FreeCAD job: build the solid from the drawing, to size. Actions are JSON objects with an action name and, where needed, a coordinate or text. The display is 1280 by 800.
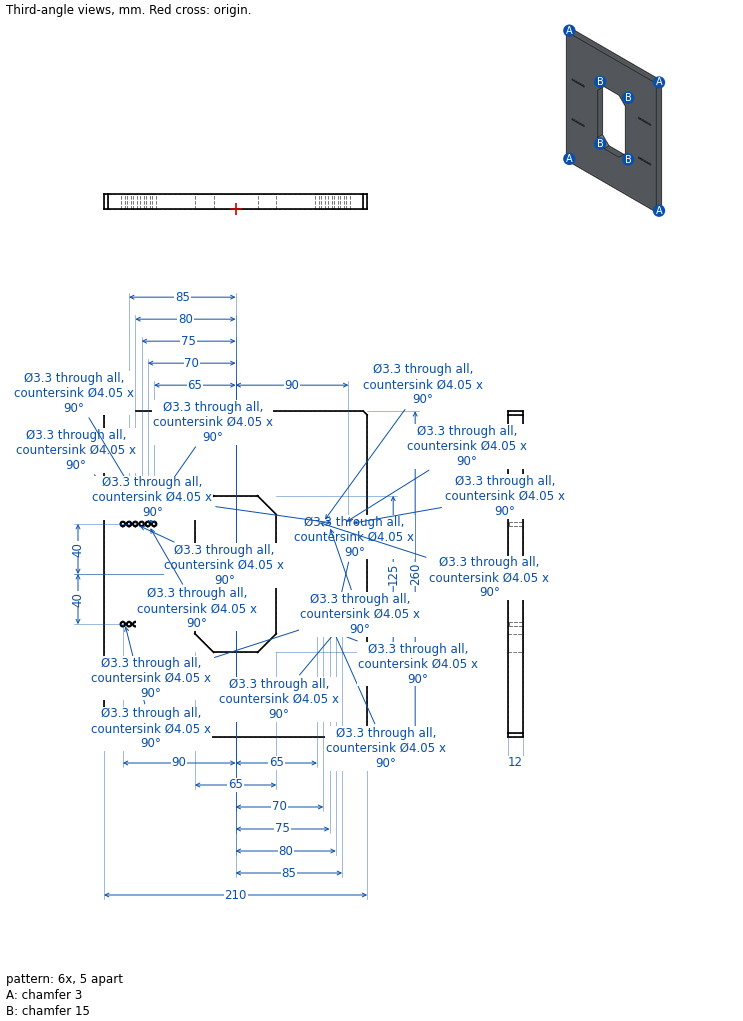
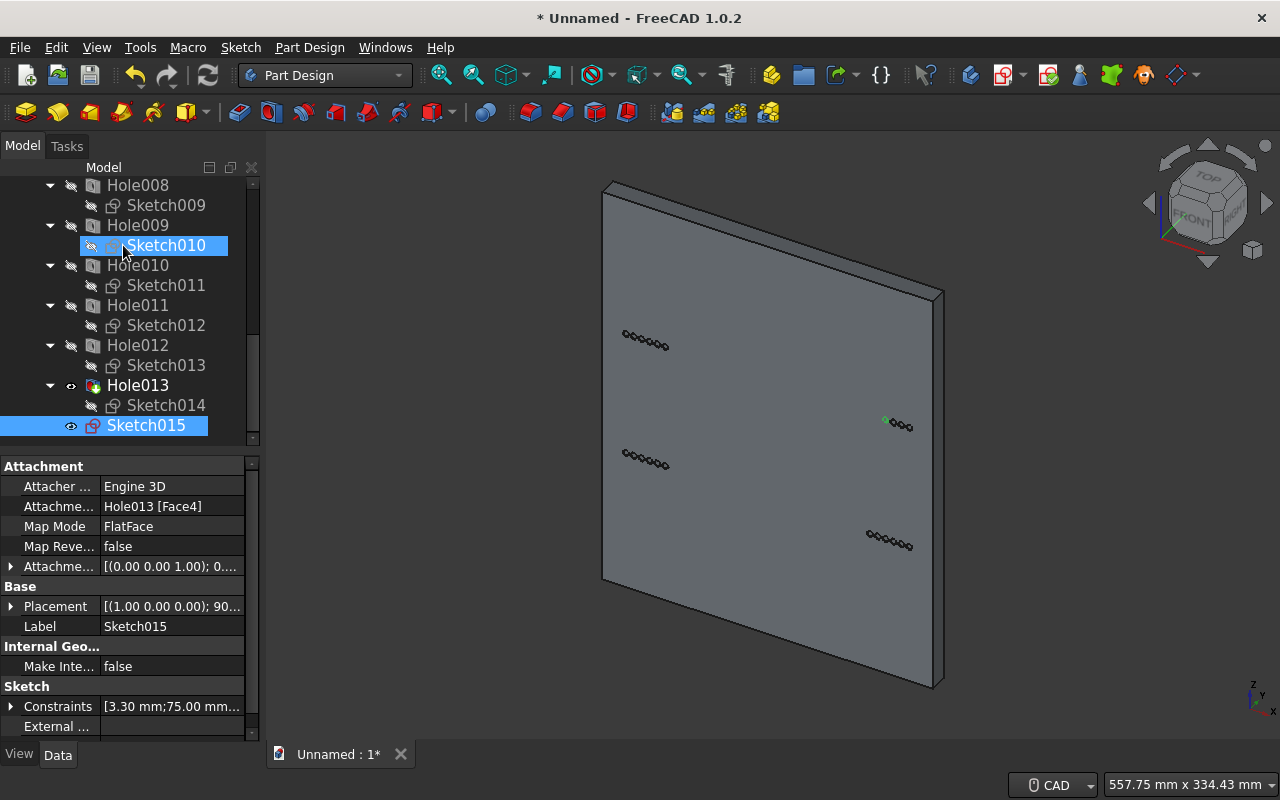
{"action": "left_click", "coordinate": [272, 112]}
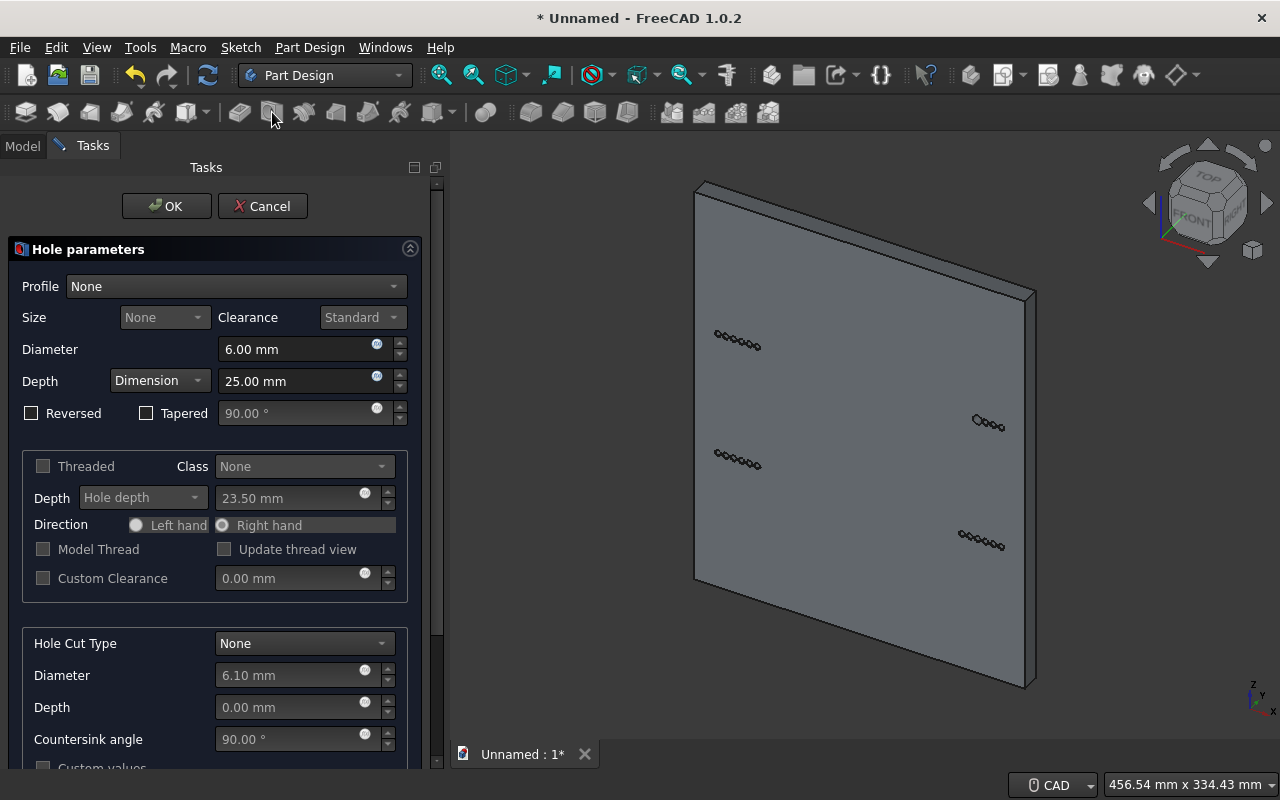
{"action": "triple_click", "coordinate": [305, 349]}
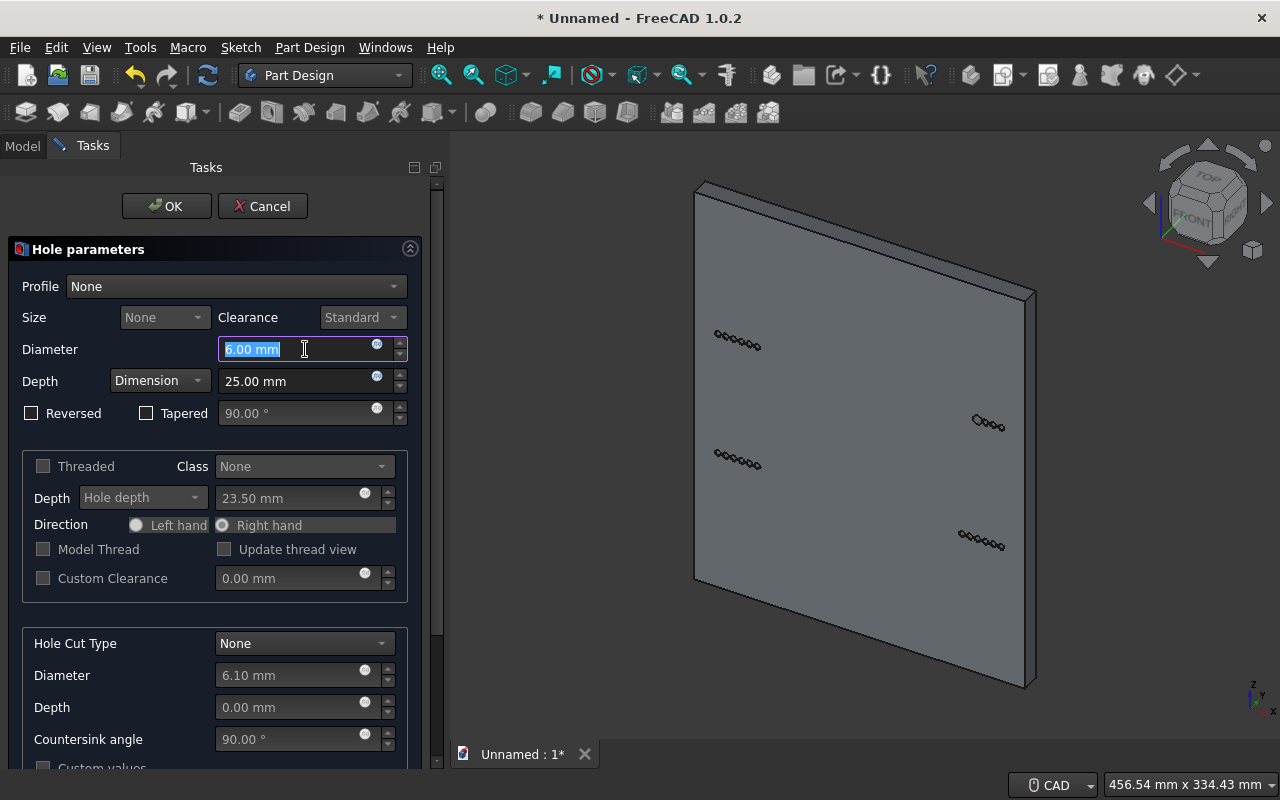
{"action": "type", "text": "3.3"}
{"action": "key", "text": "Tab"}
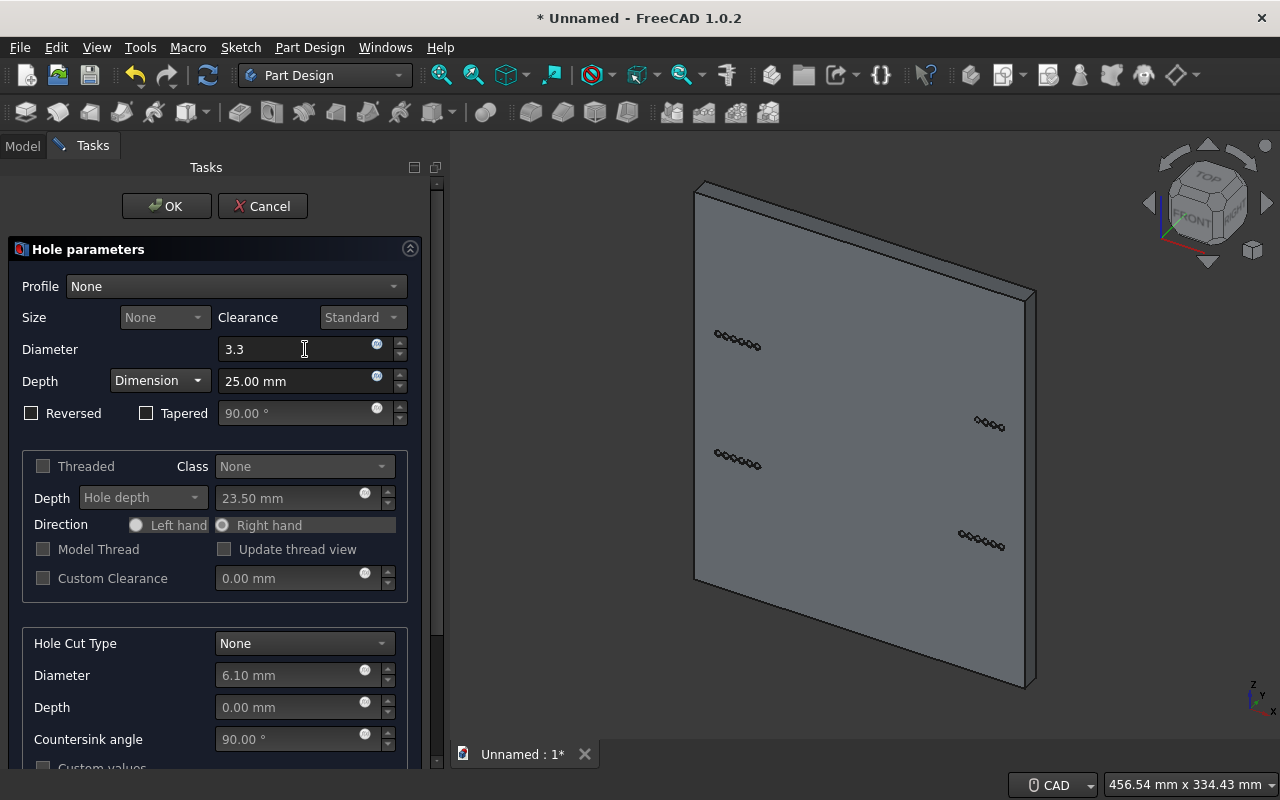
{"action": "left_click", "coordinate": [161, 380]}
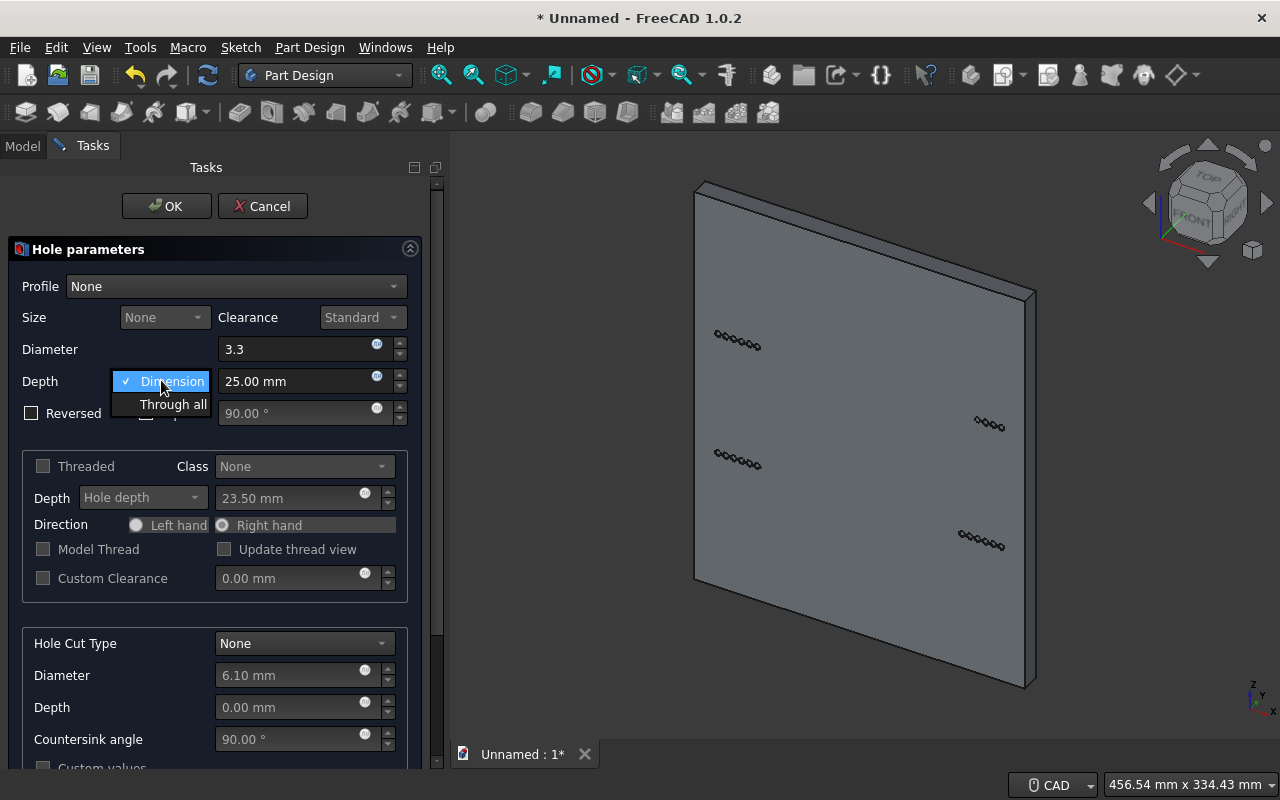
{"action": "left_click", "coordinate": [160, 404]}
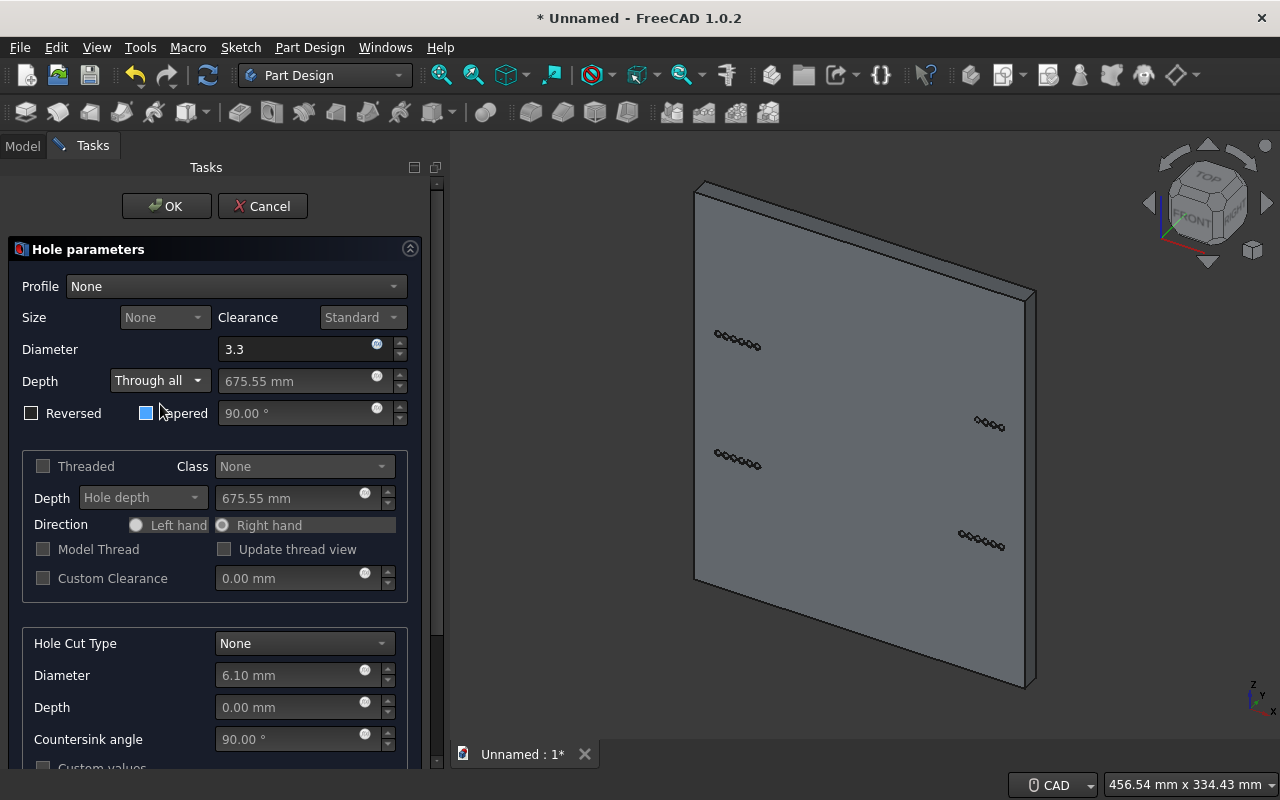
{"action": "left_click", "coordinate": [306, 644]}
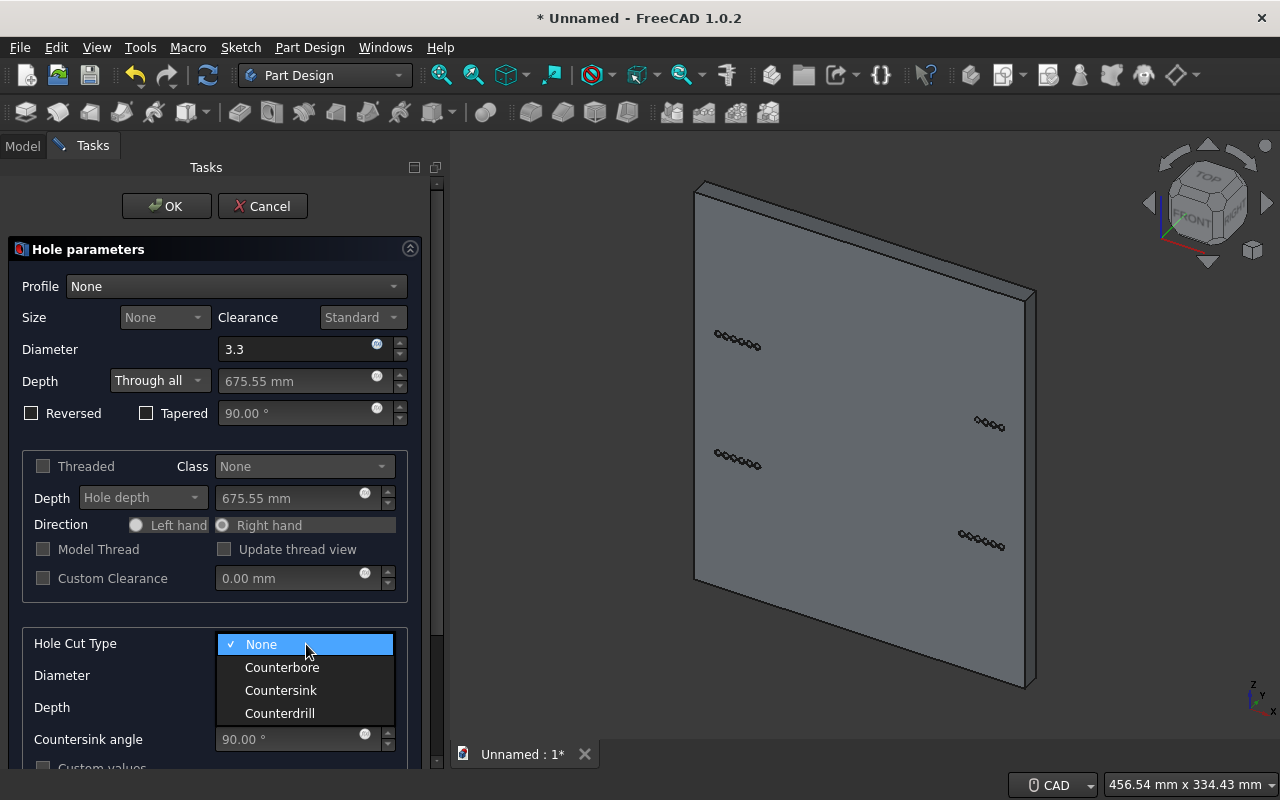
{"action": "left_click", "coordinate": [304, 690]}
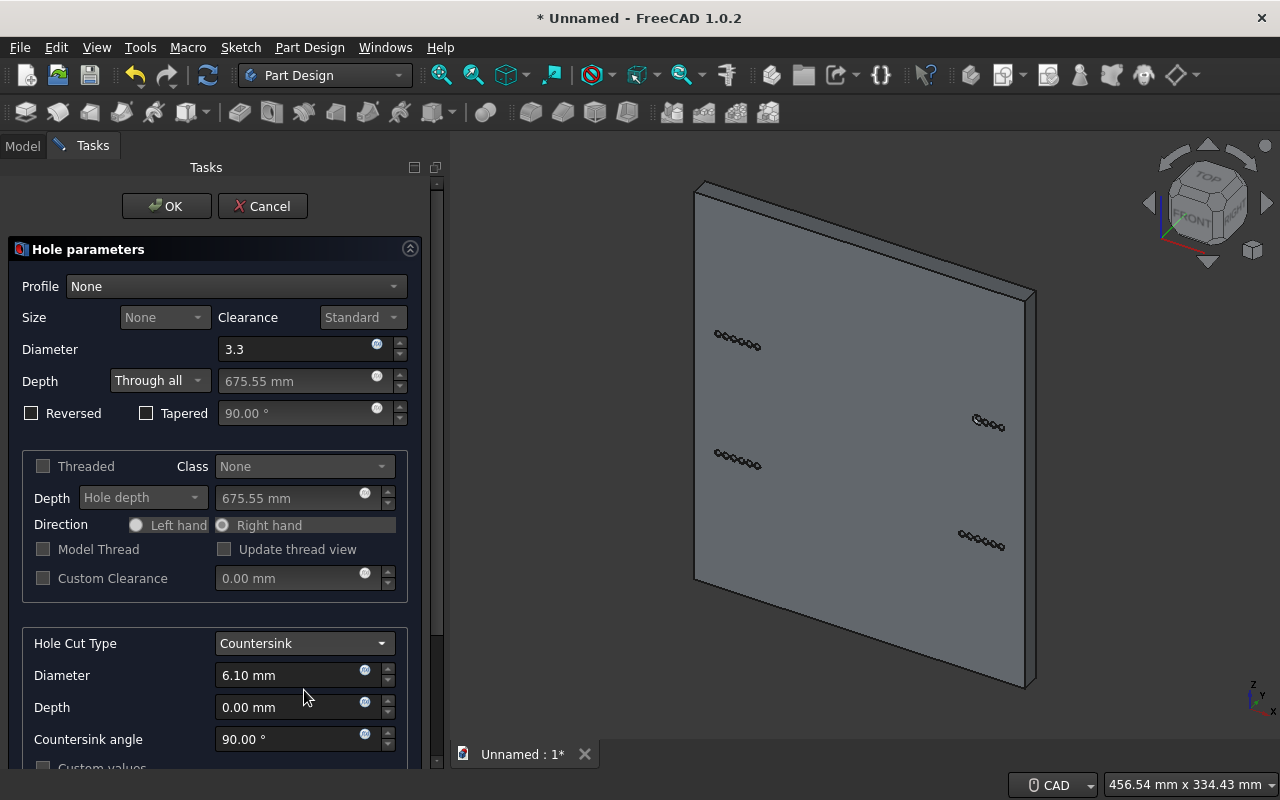
{"action": "triple_click", "coordinate": [298, 675]}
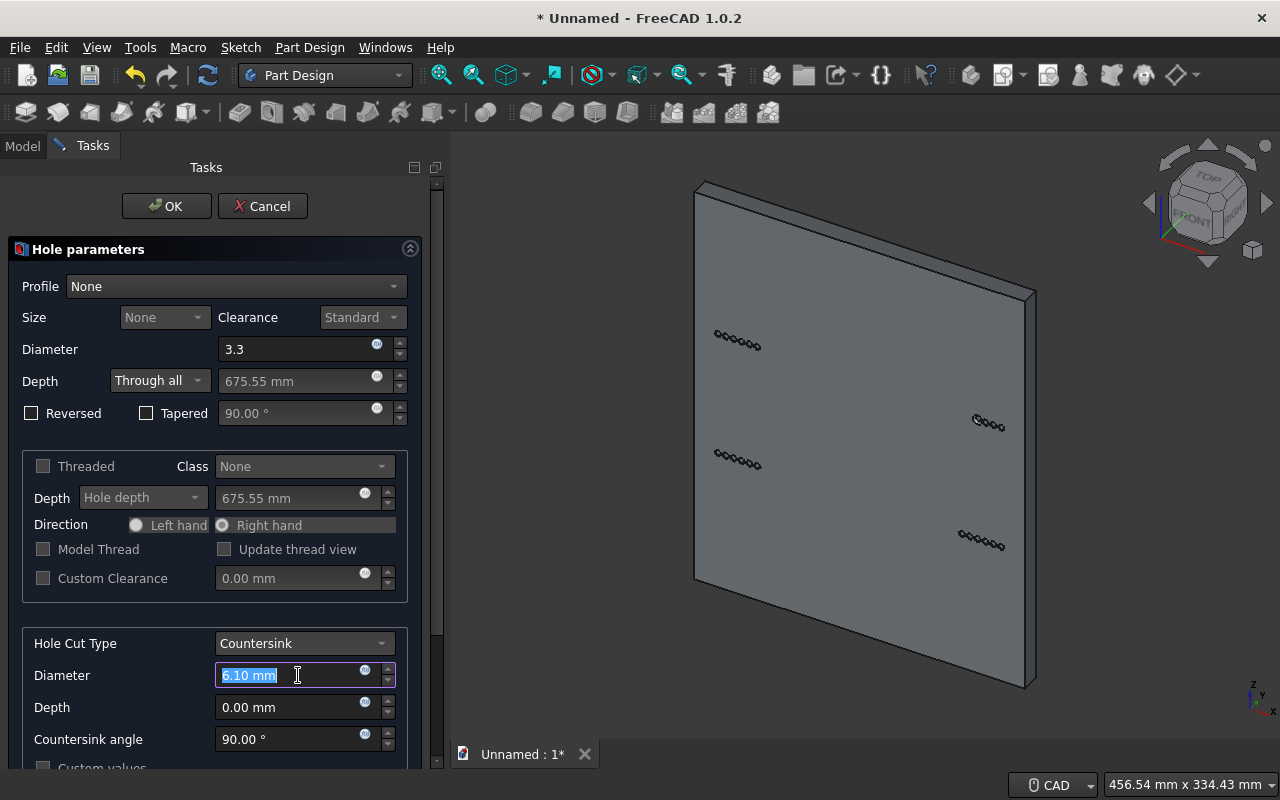
{"action": "type", "text": "4.05"}
{"action": "key", "text": "Tab"}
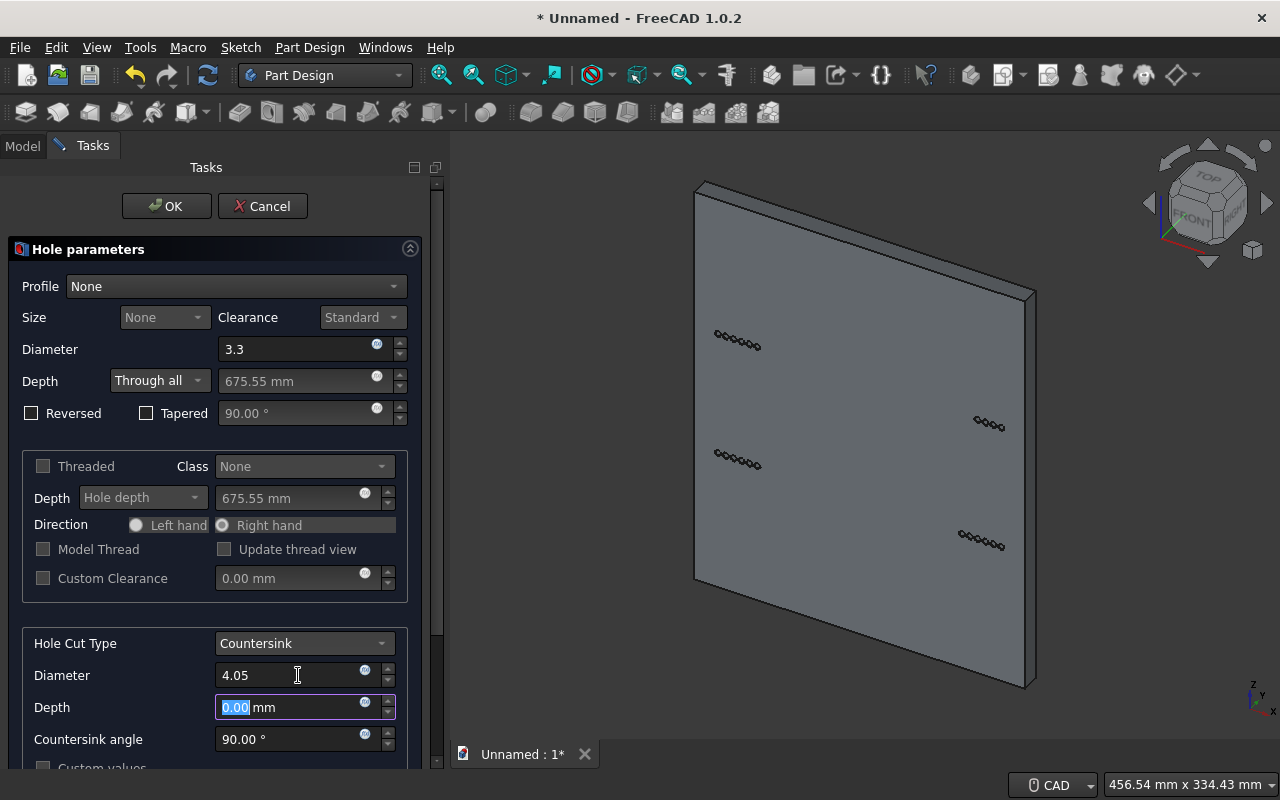
{"action": "left_click", "coordinate": [167, 206]}